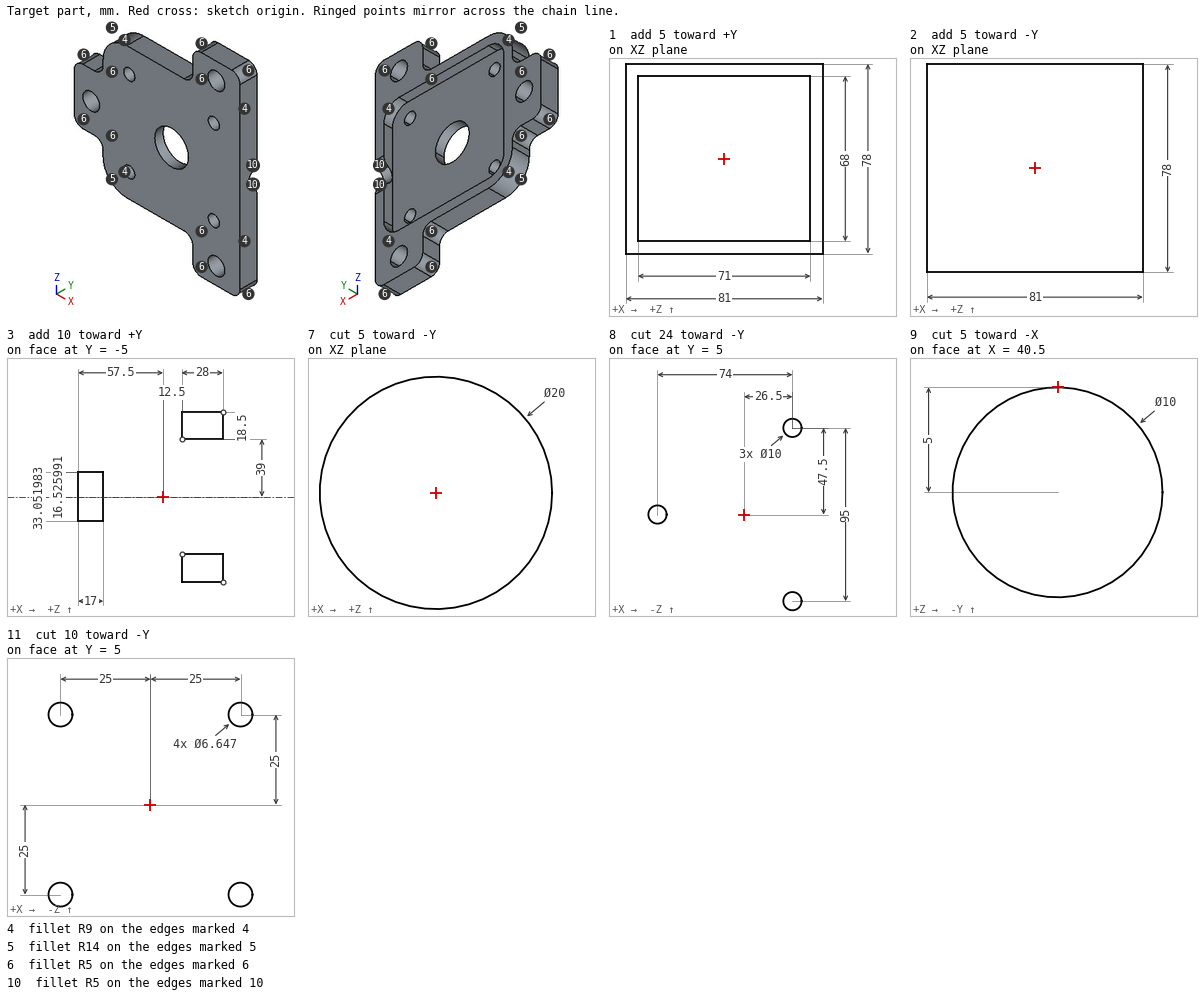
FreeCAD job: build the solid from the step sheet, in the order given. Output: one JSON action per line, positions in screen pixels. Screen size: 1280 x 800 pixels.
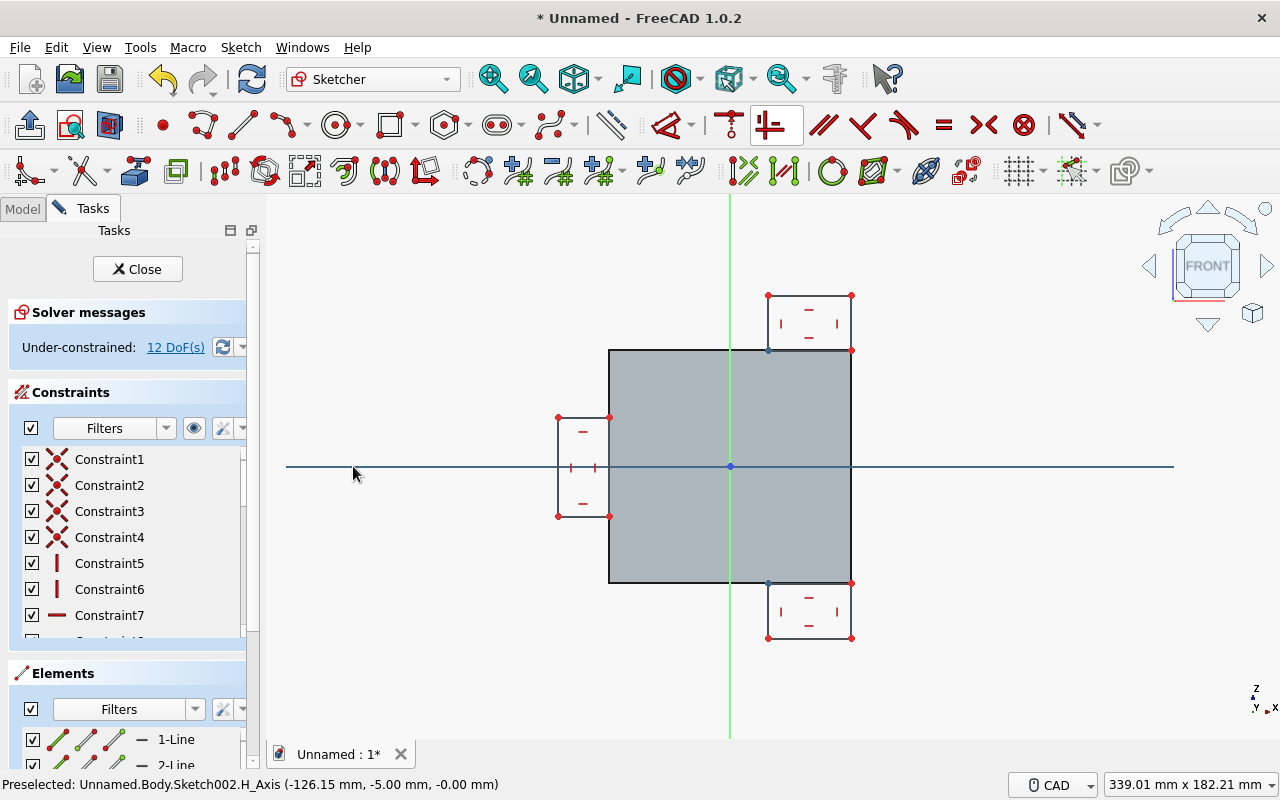
{"action": "key", "text": "s"}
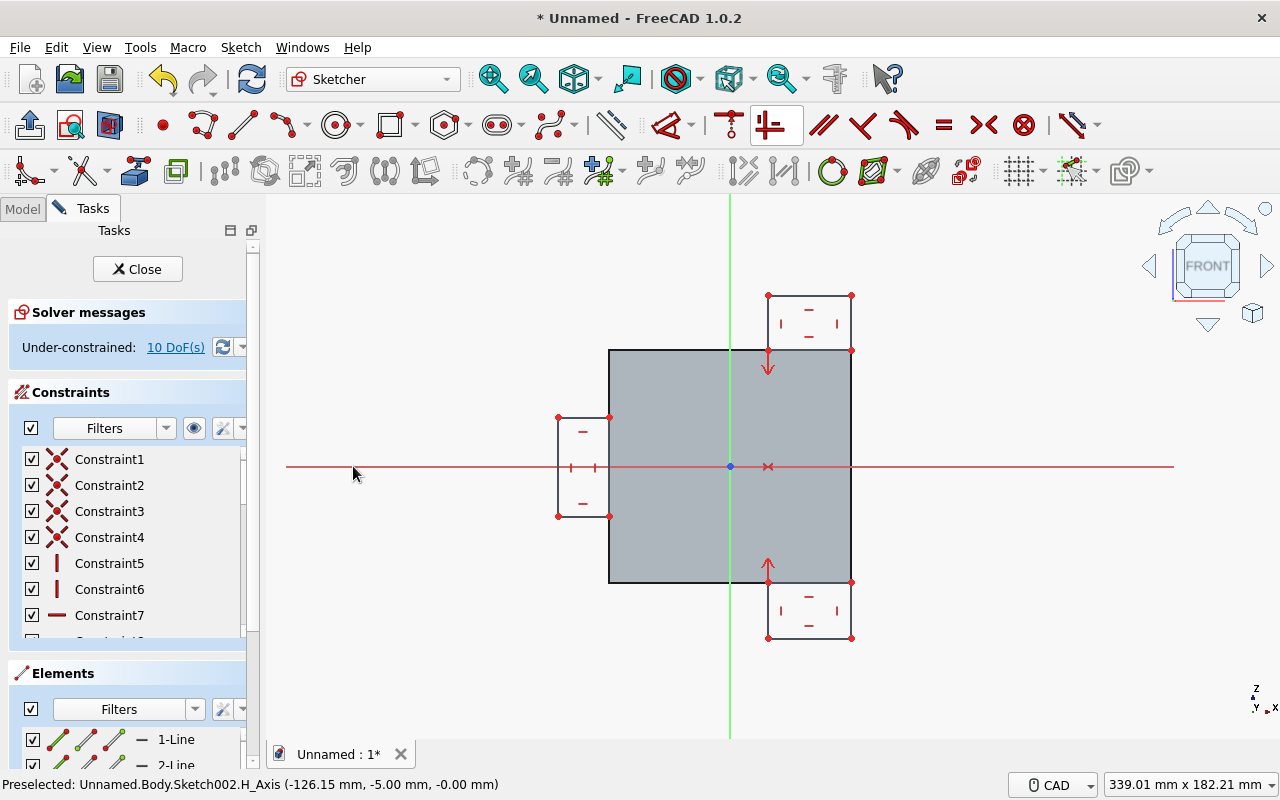
{"action": "left_click", "coordinate": [851, 296]}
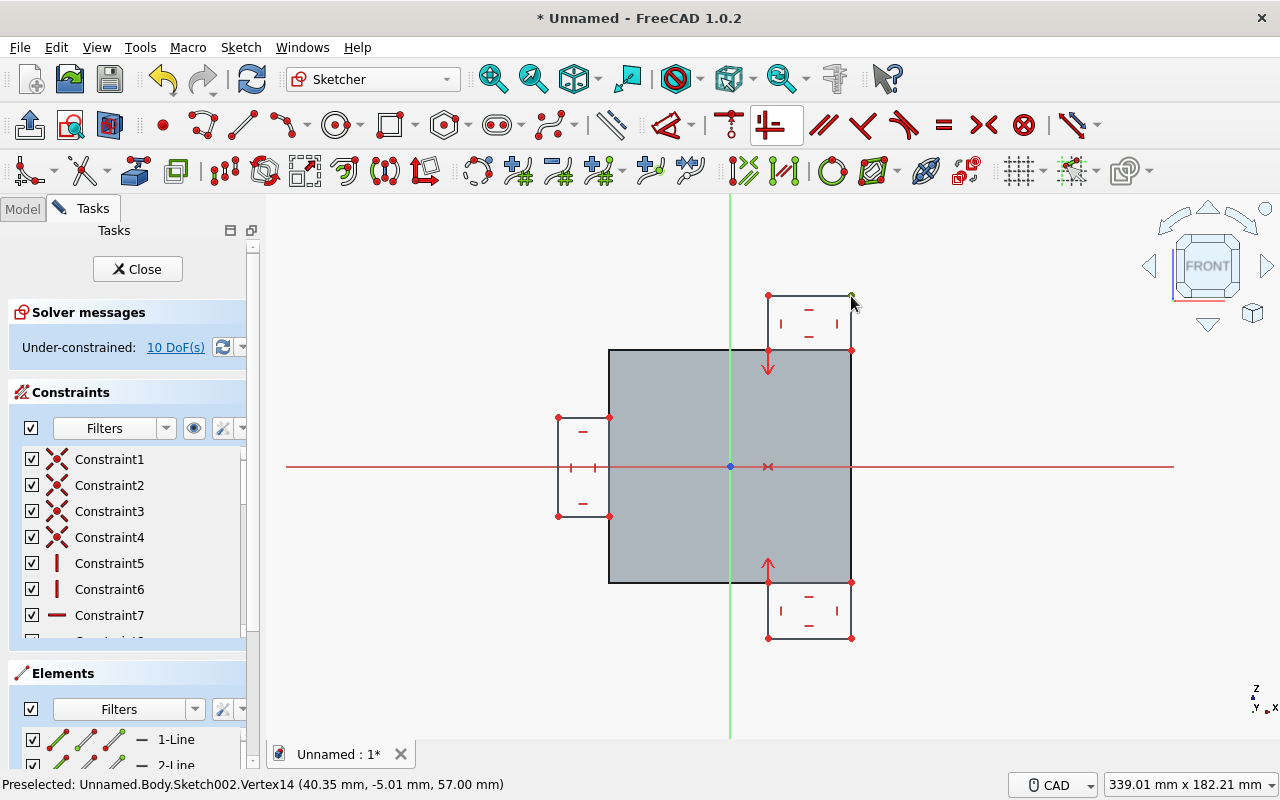
{"action": "left_click", "coordinate": [851, 639]}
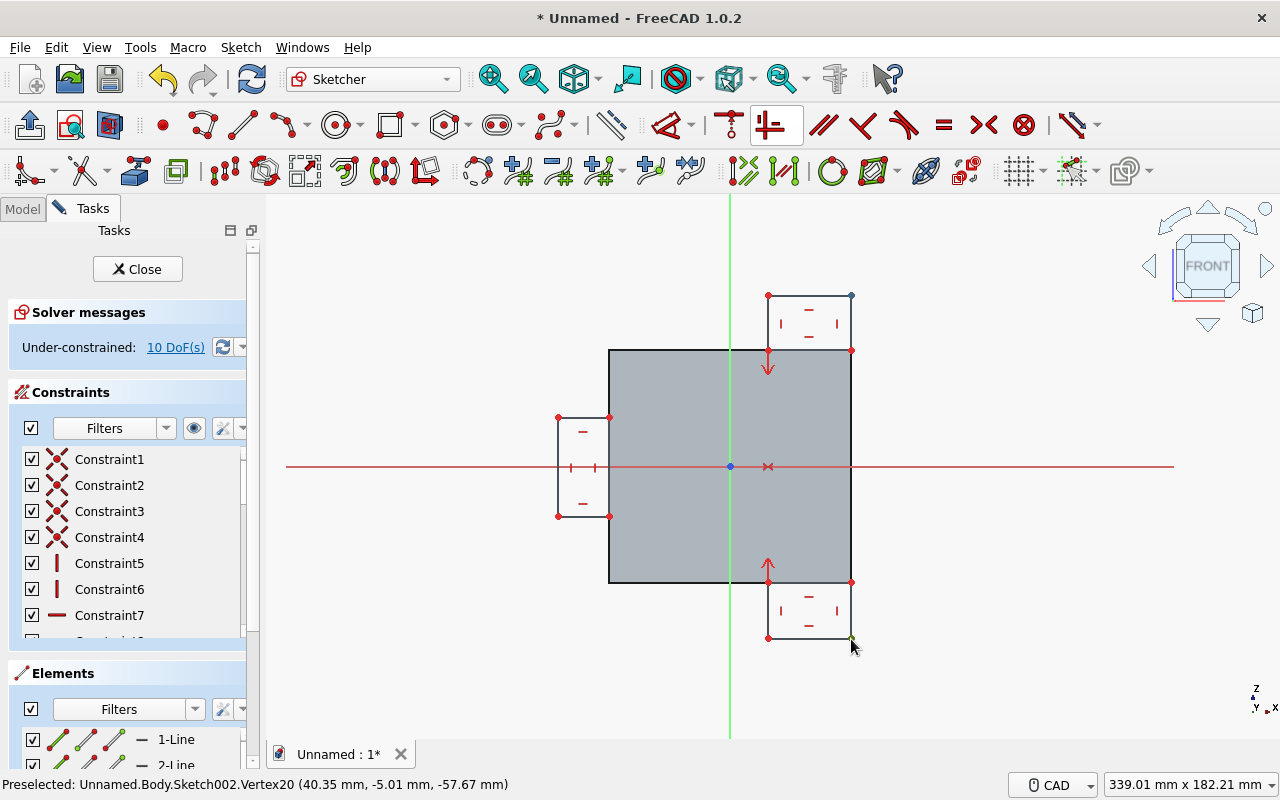
{"action": "left_click", "coordinate": [353, 466]}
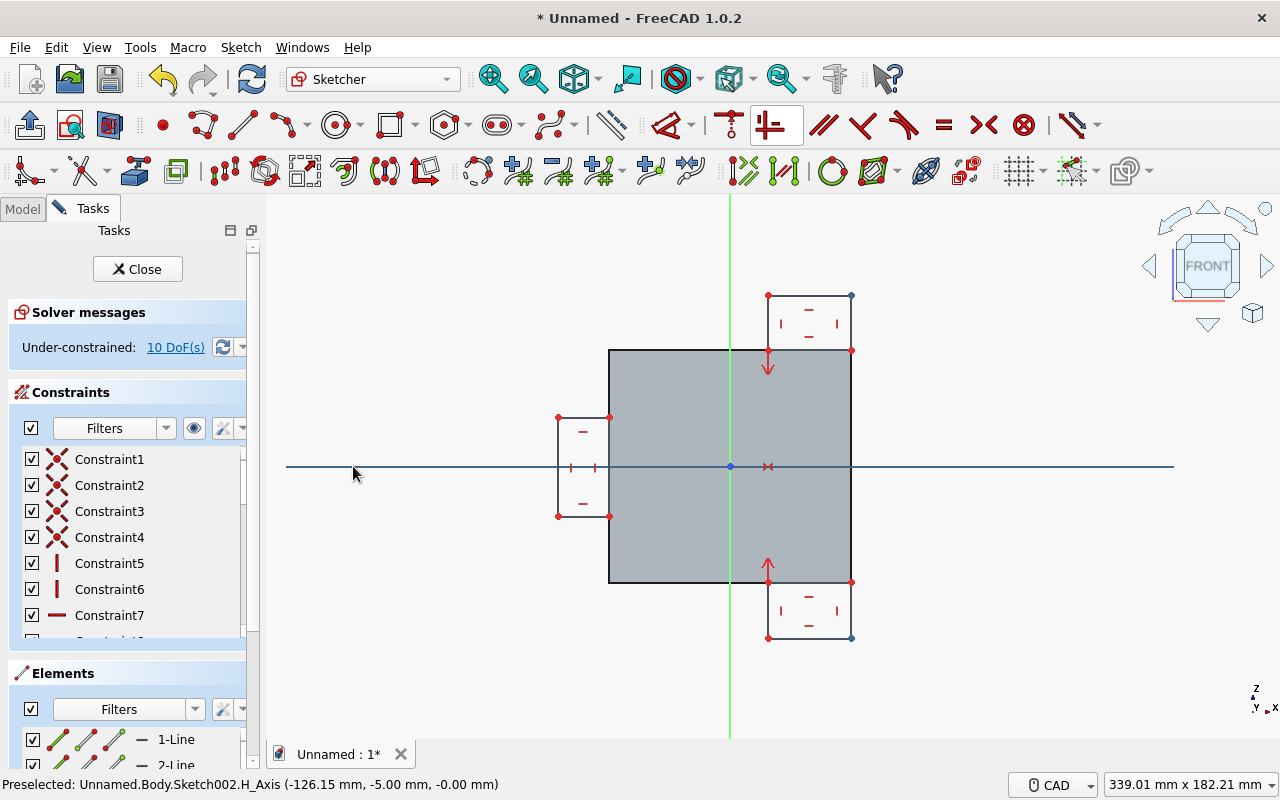
{"action": "left_click", "coordinate": [984, 126]}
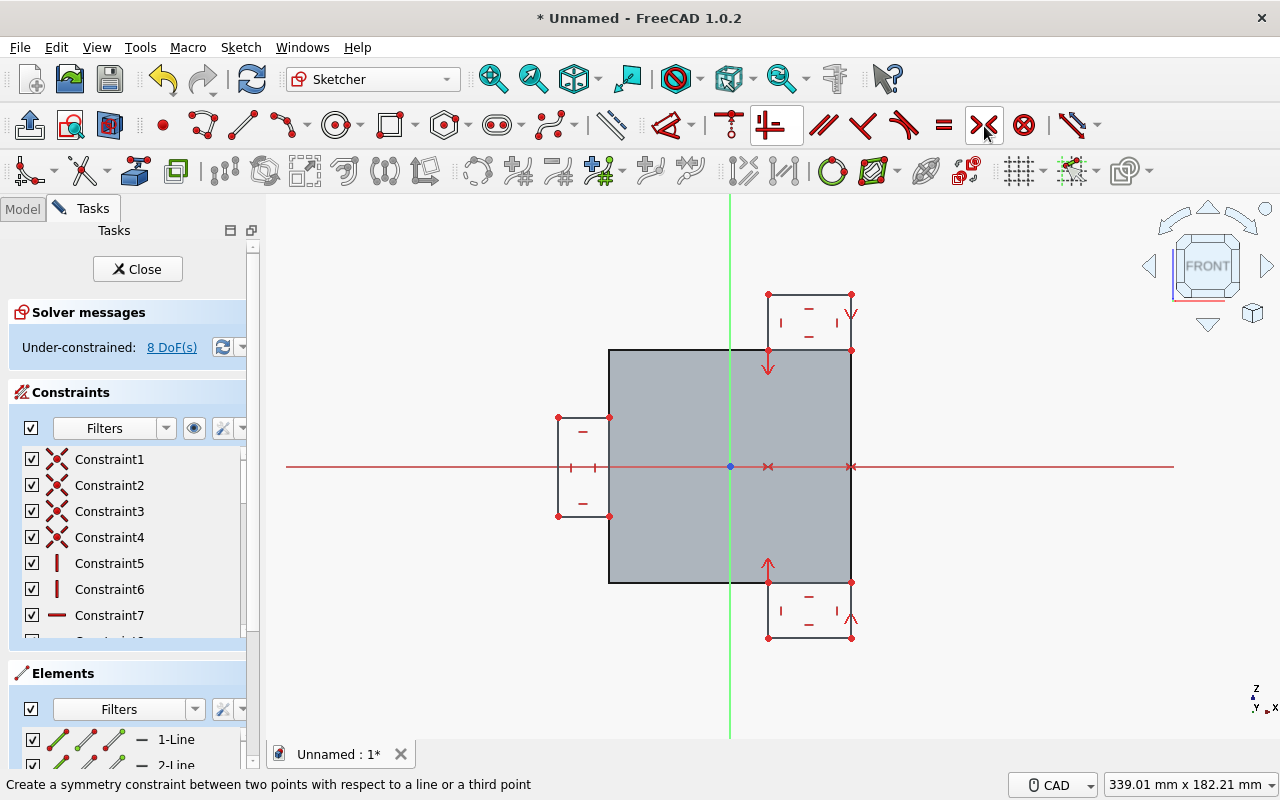
{"action": "left_click", "coordinate": [666, 126]}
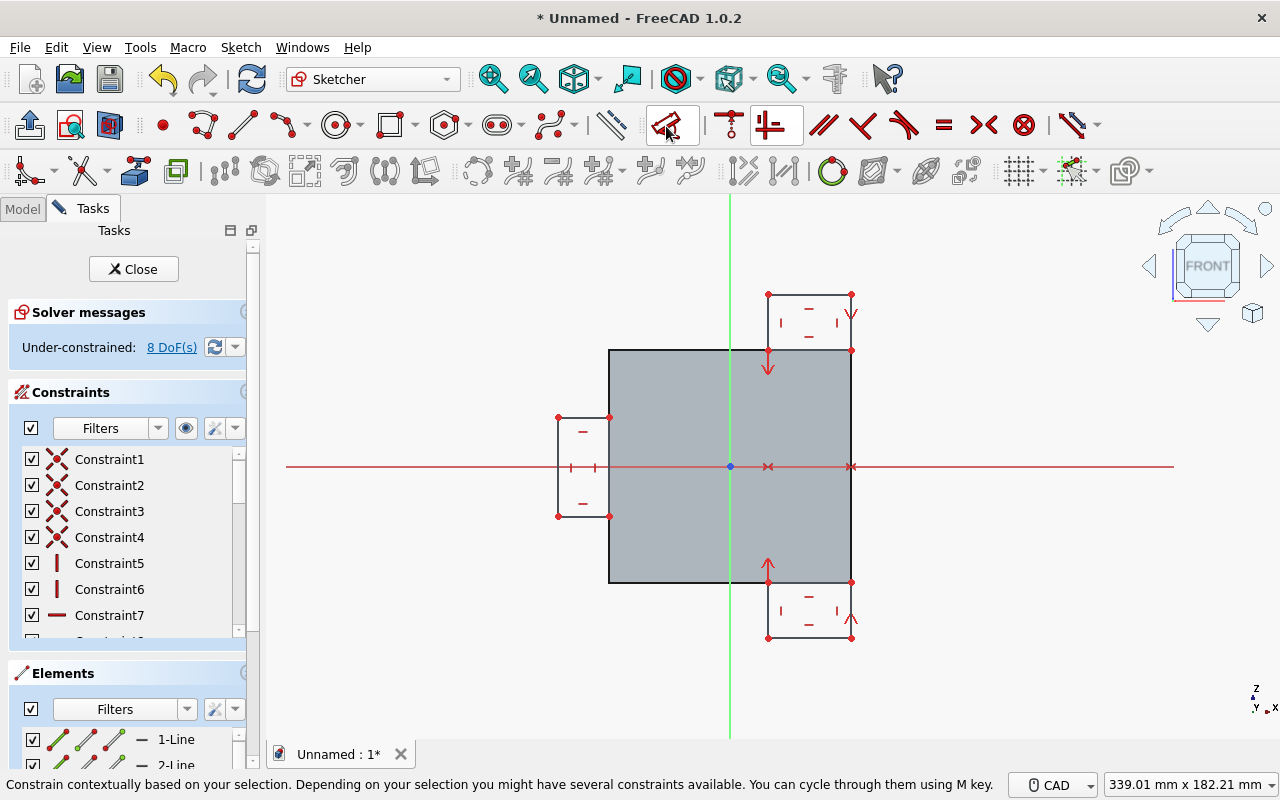
{"action": "left_click", "coordinate": [573, 517]}
{"action": "left_click", "coordinate": [583, 551]}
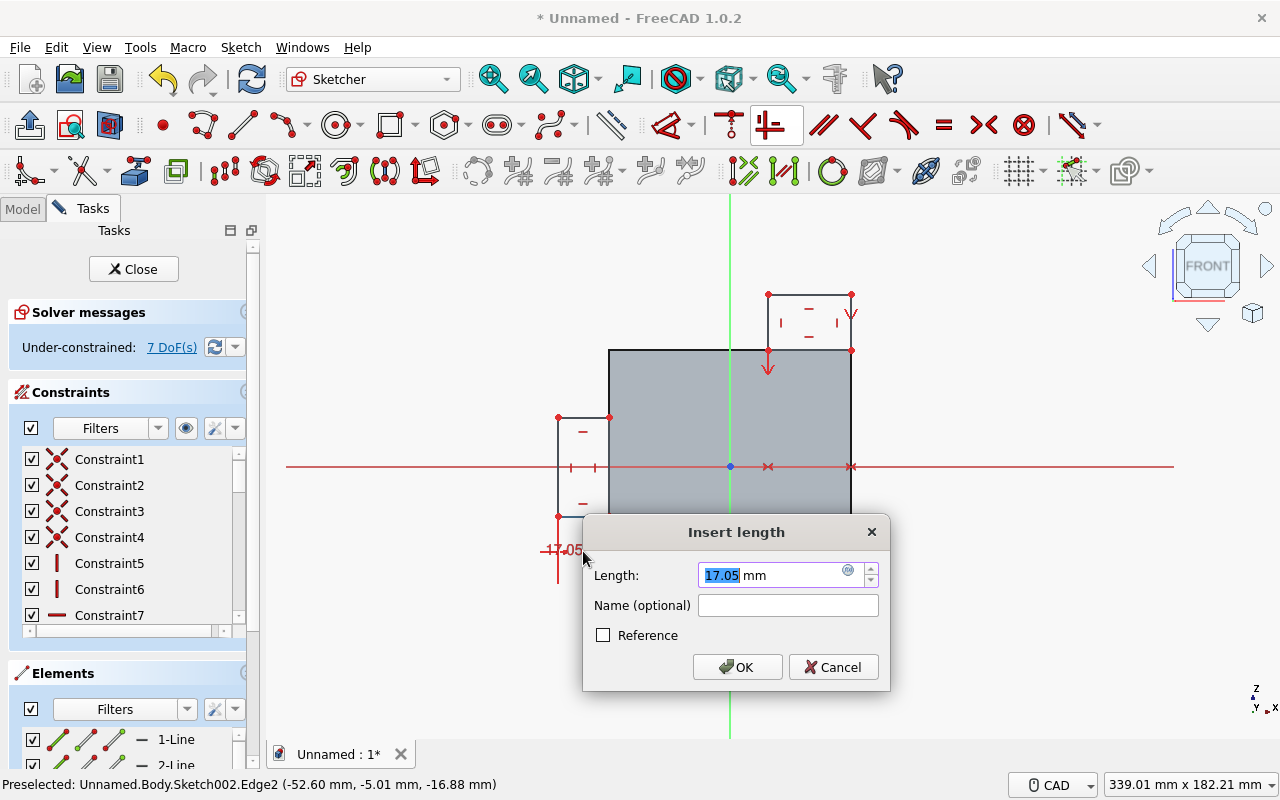
{"action": "type", "text": "17"}
{"action": "key", "text": "Return"}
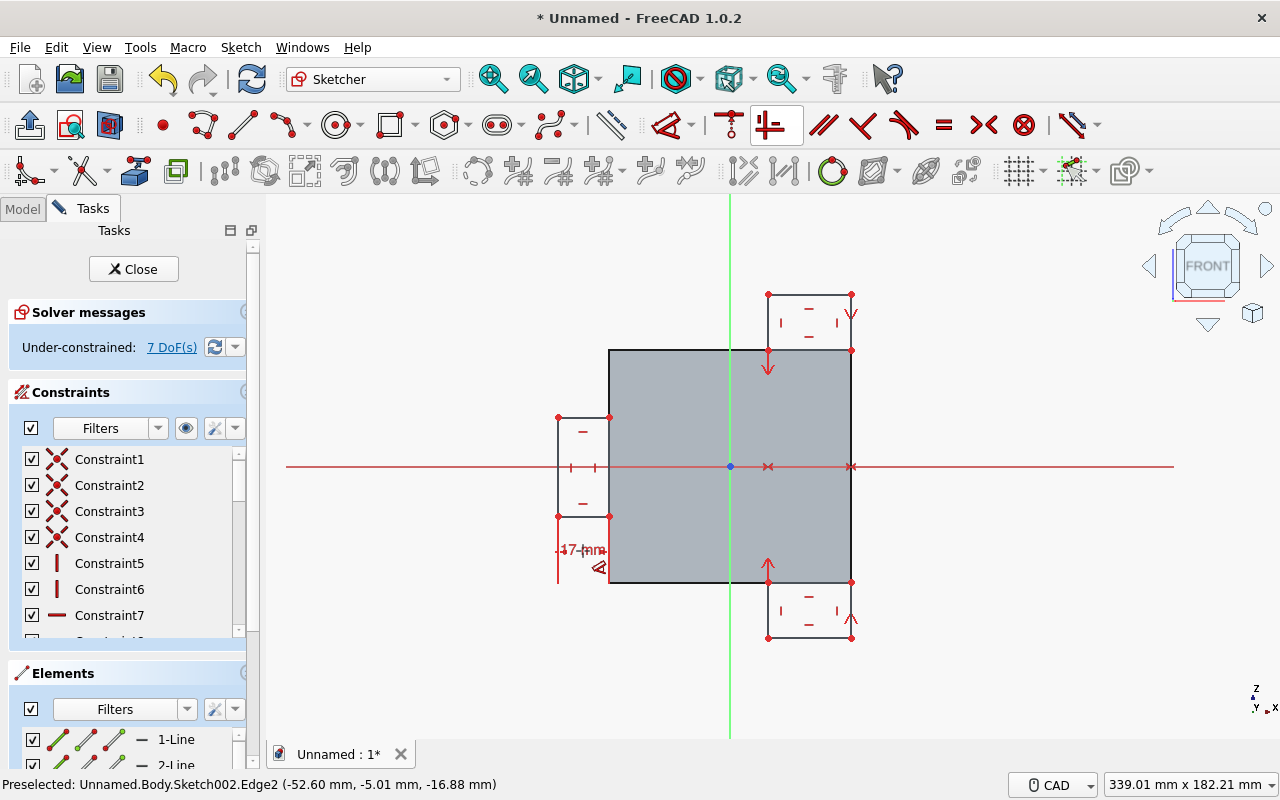
{"action": "left_click", "coordinate": [793, 350]}
{"action": "left_click", "coordinate": [810, 316]}